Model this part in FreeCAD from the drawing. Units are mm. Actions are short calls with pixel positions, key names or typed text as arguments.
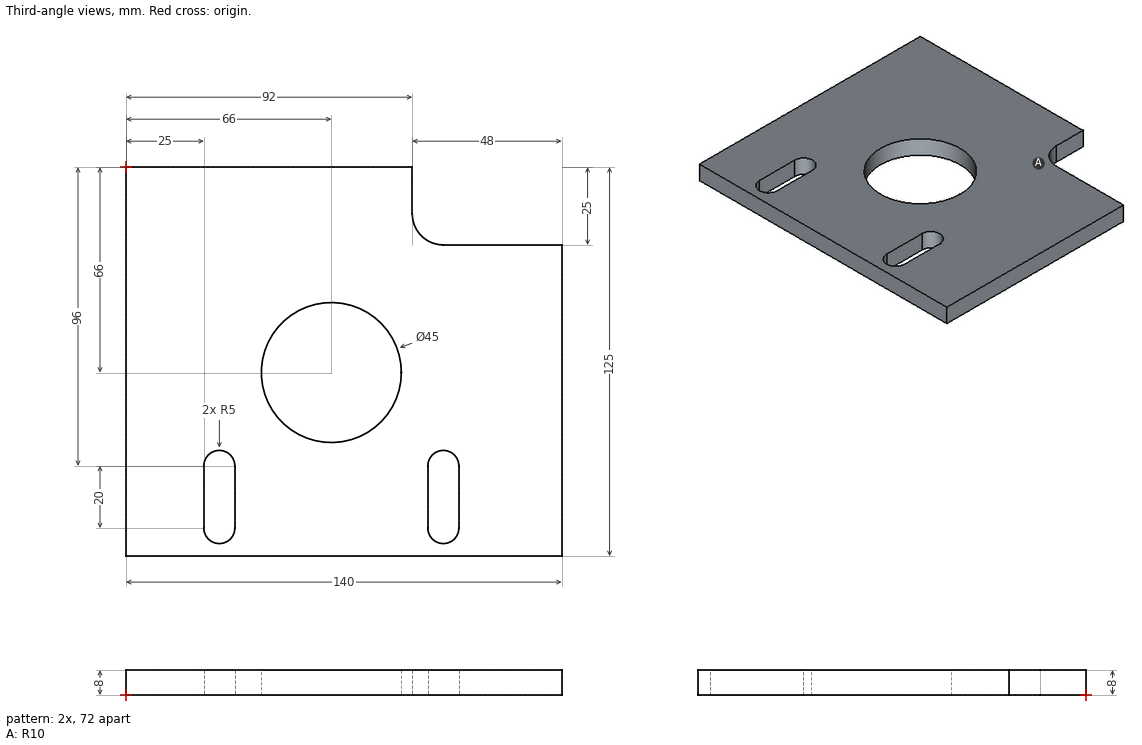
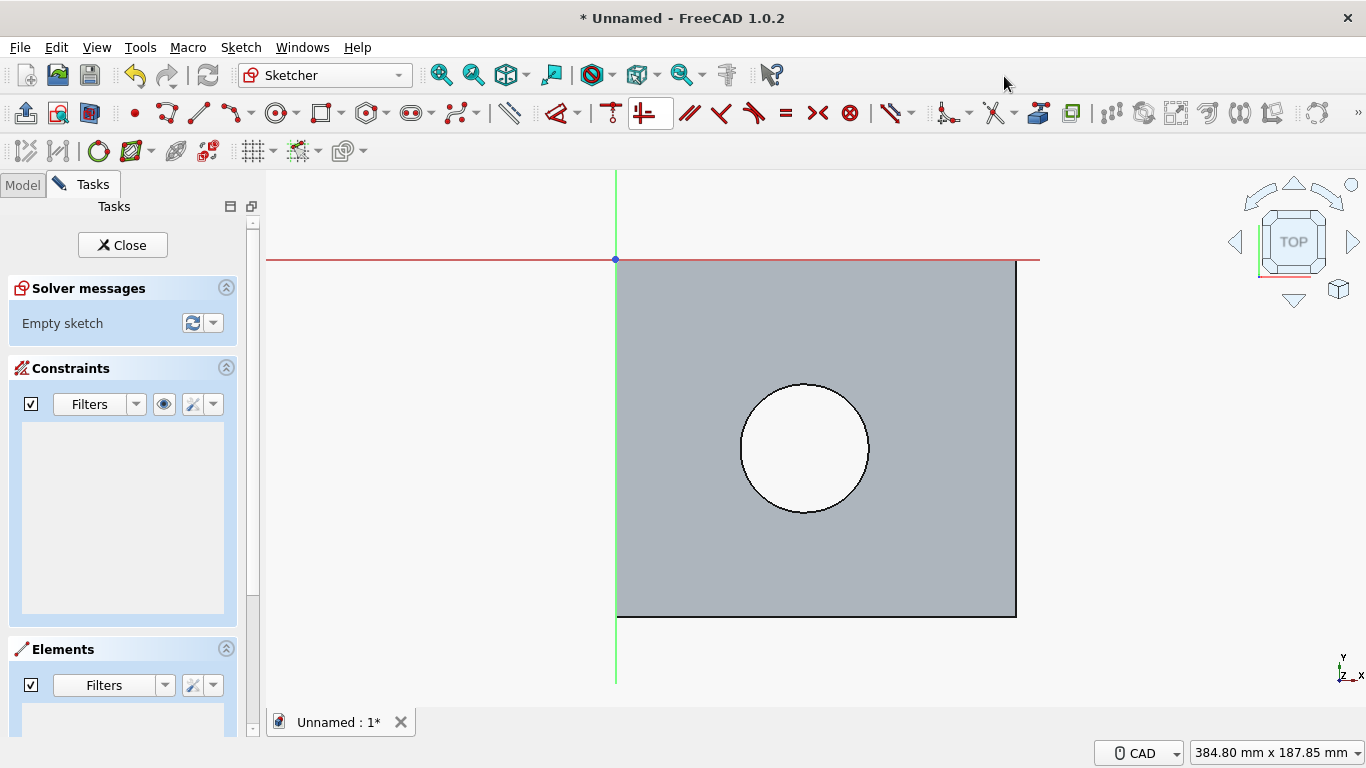
scroll(687, 604, up, 7)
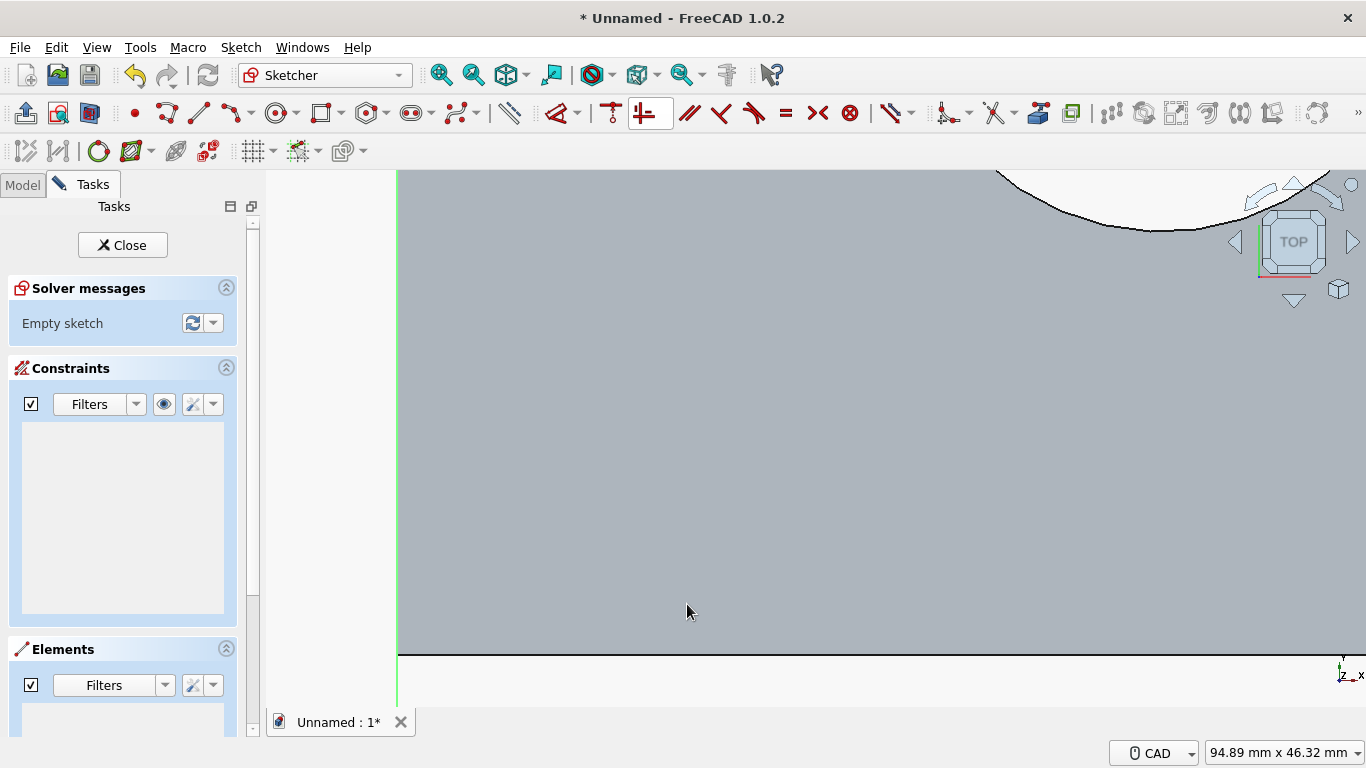
click(412, 114)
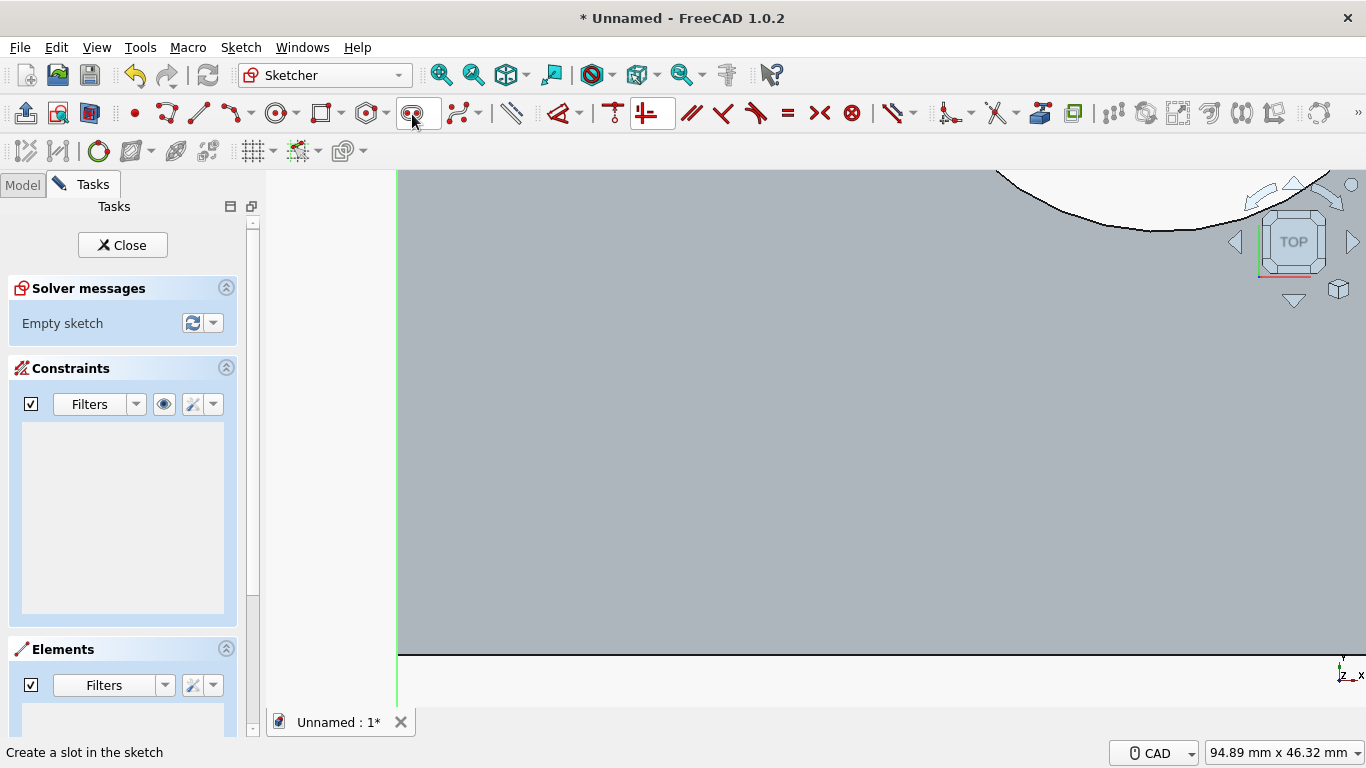
click(745, 551)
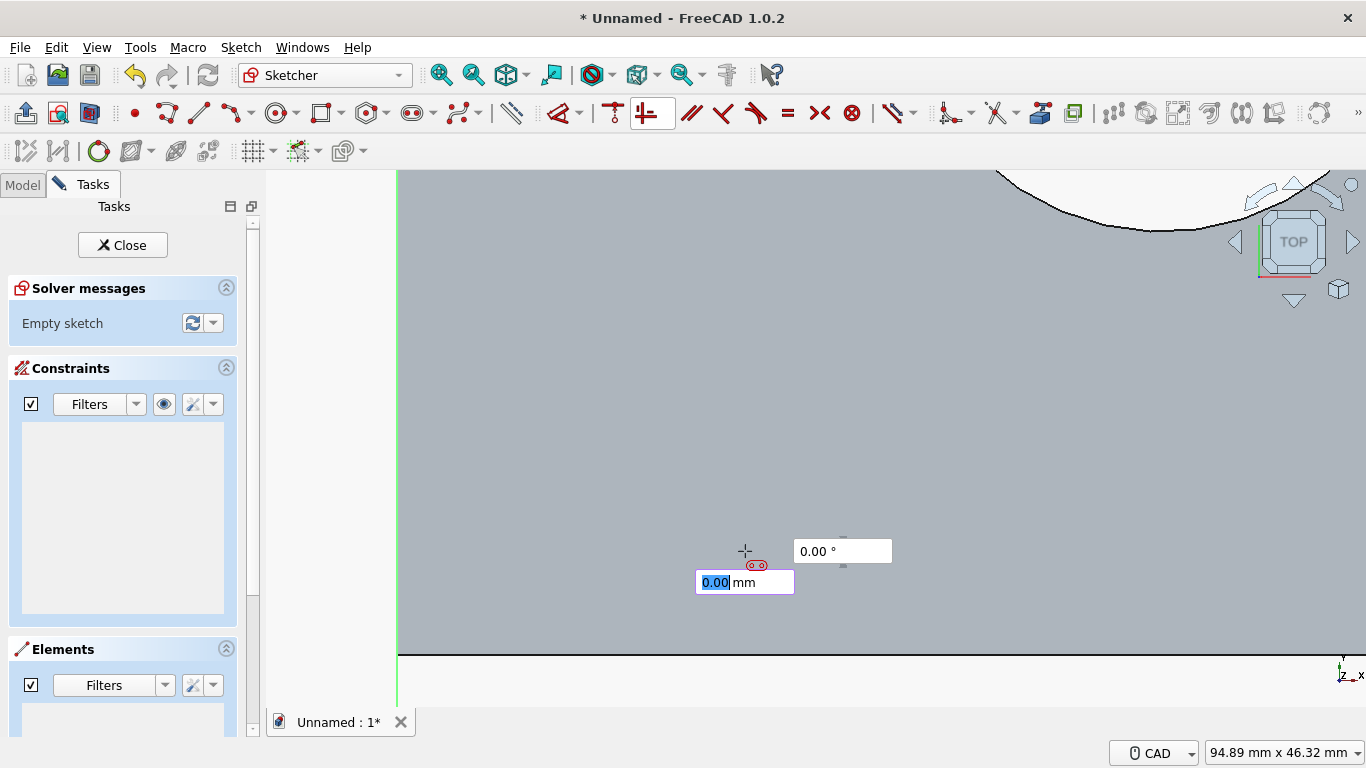
click(745, 319)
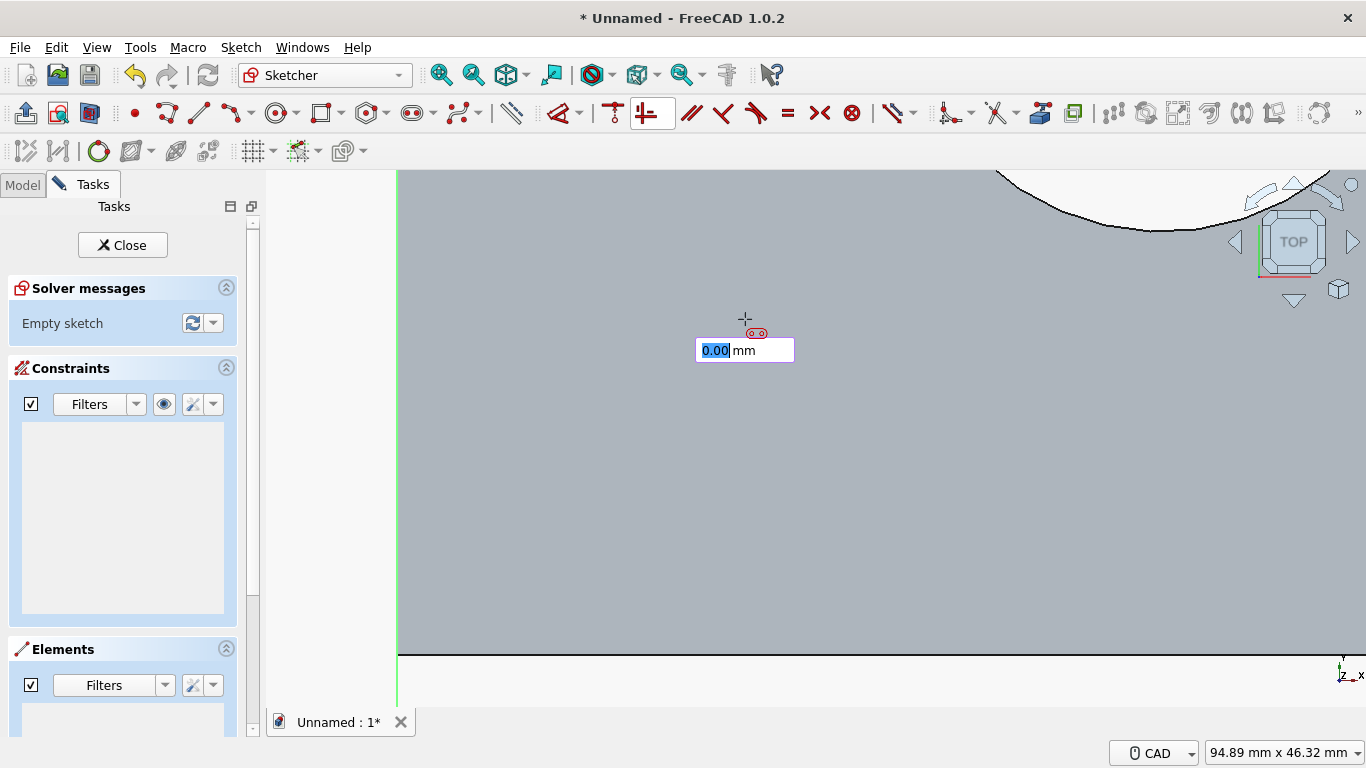
click(803, 435)
key(Escape)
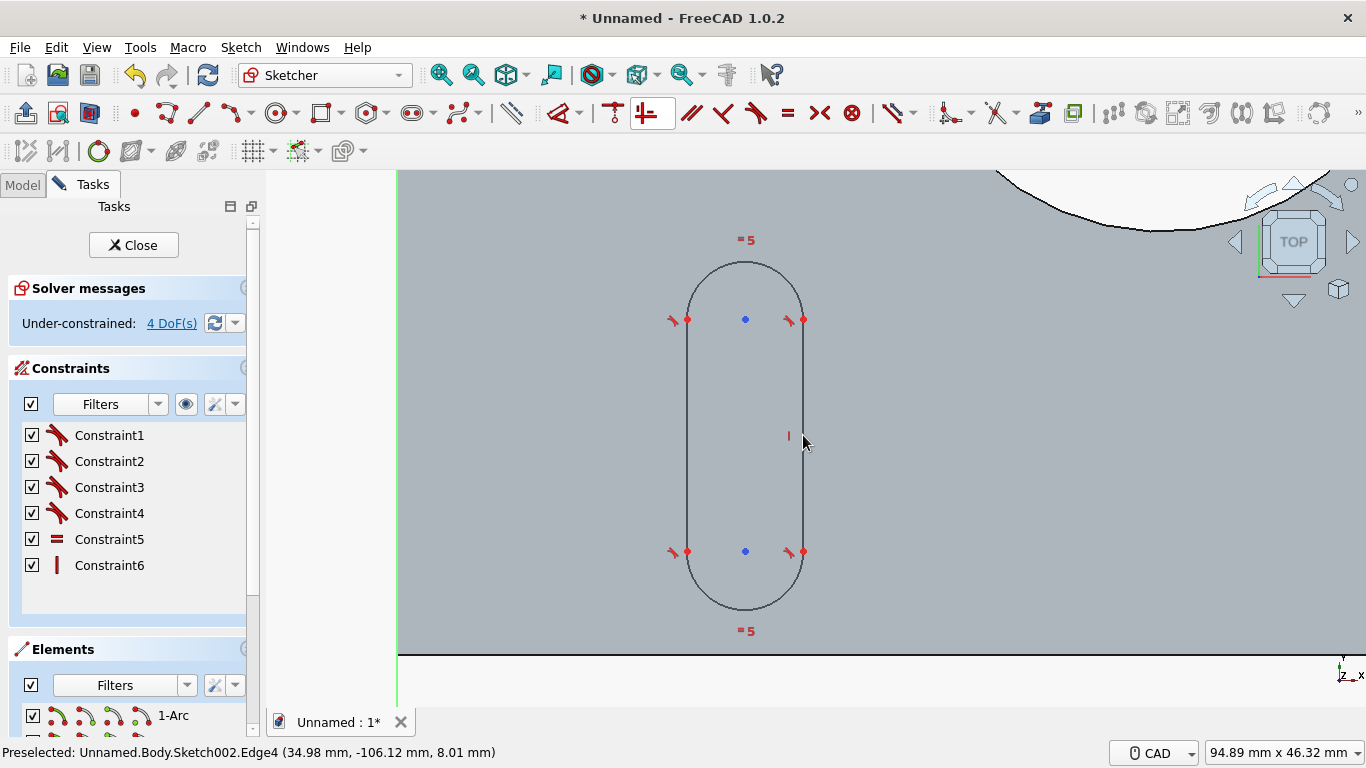
click(711, 599)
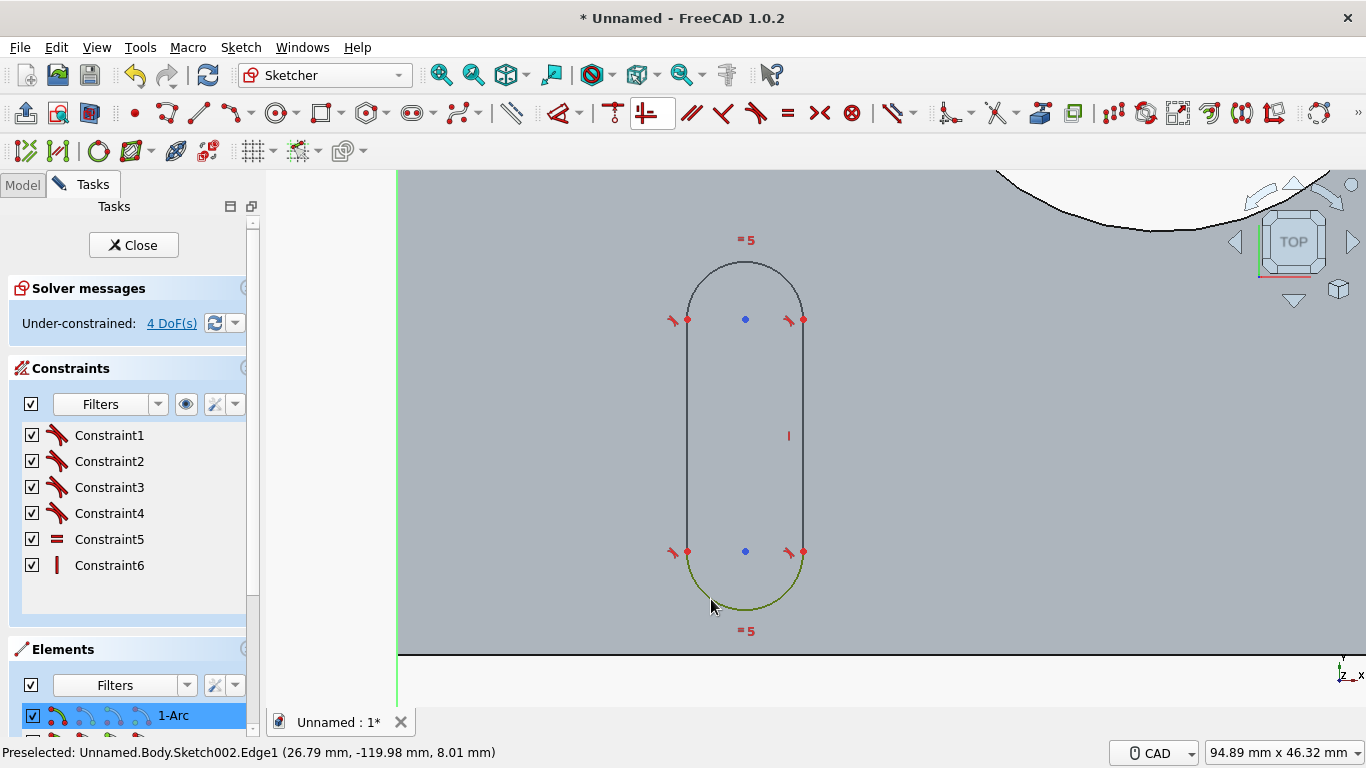
key(k)
key(r)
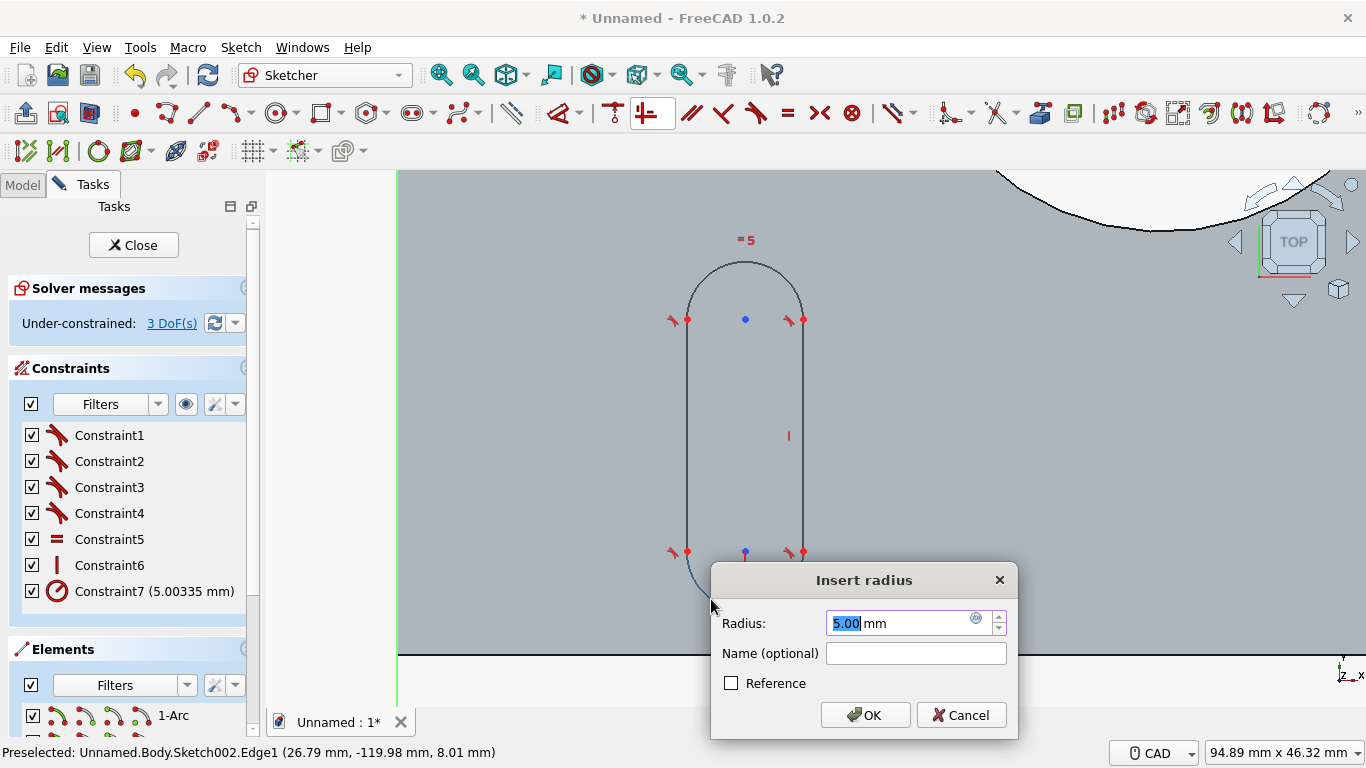
text(5)
key(Return)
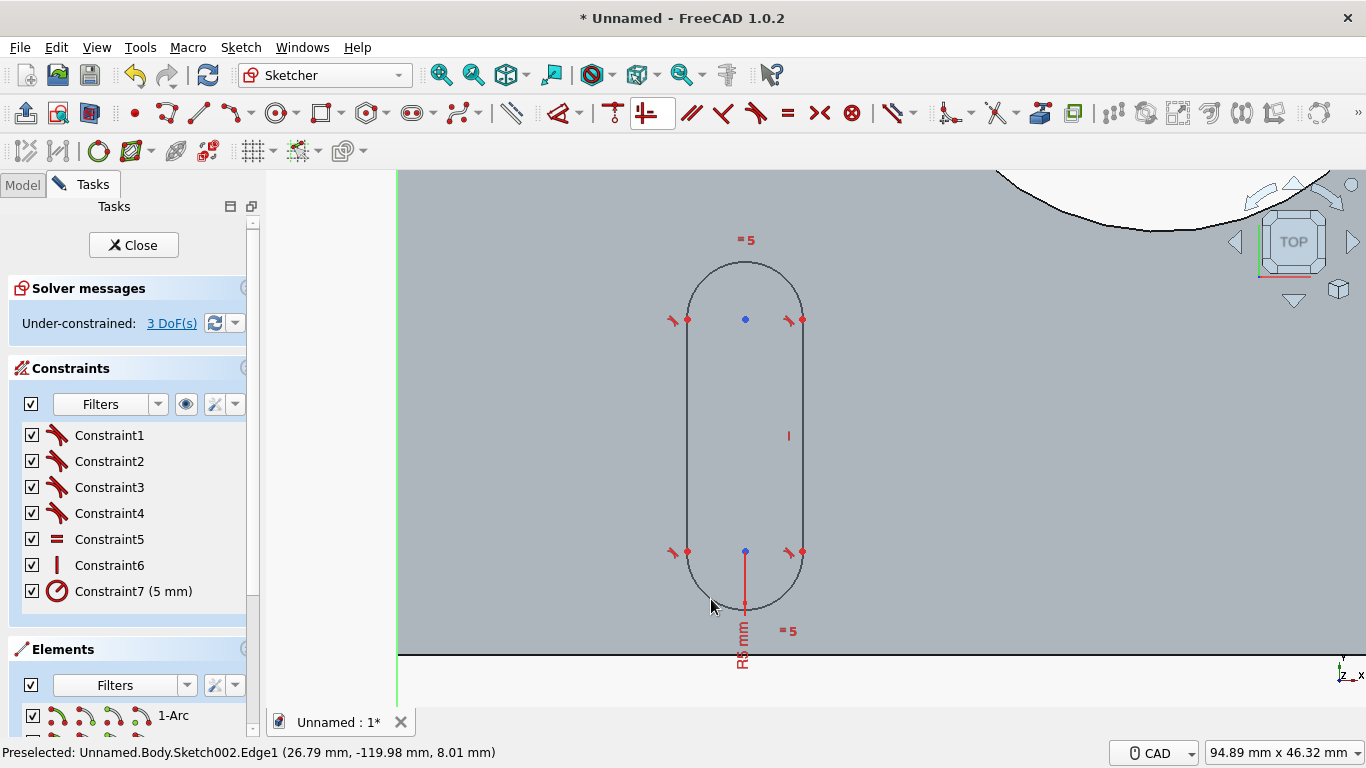
click(687, 482)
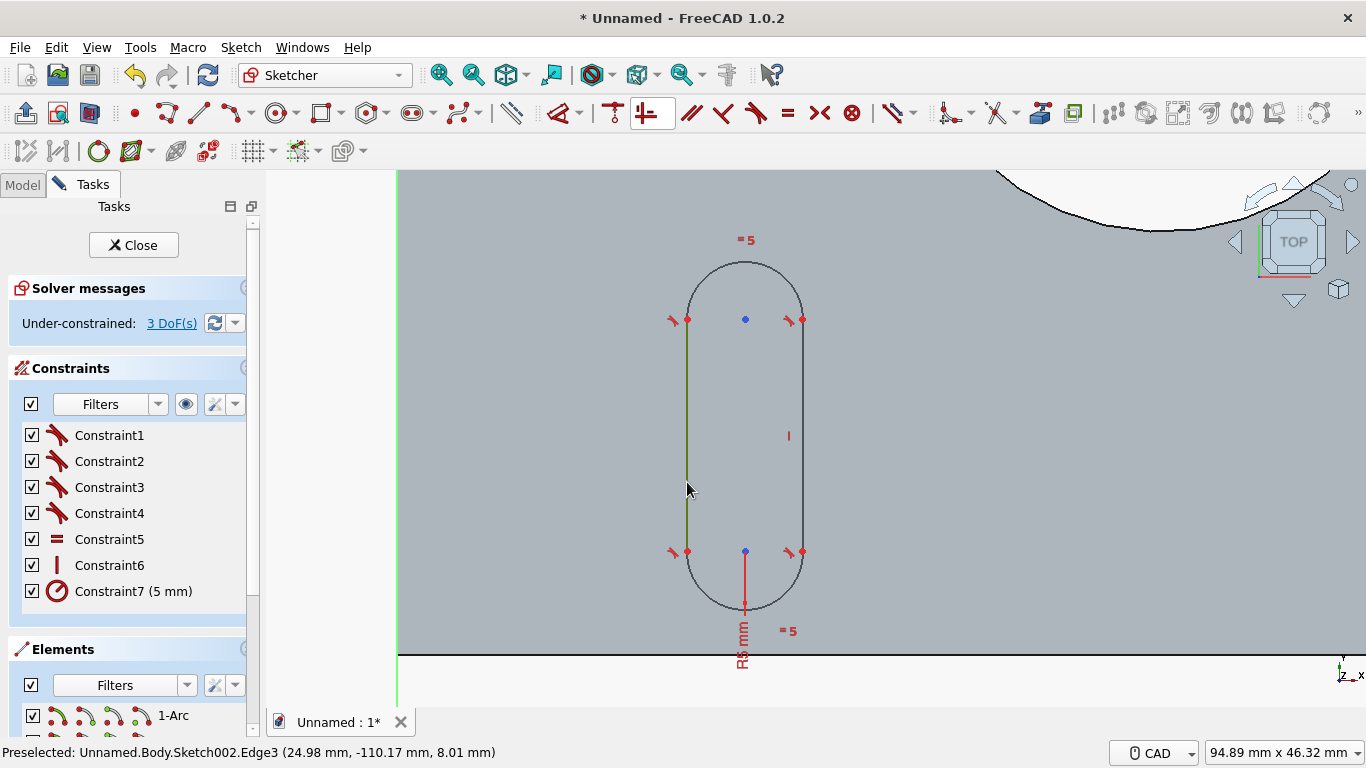
key(i)